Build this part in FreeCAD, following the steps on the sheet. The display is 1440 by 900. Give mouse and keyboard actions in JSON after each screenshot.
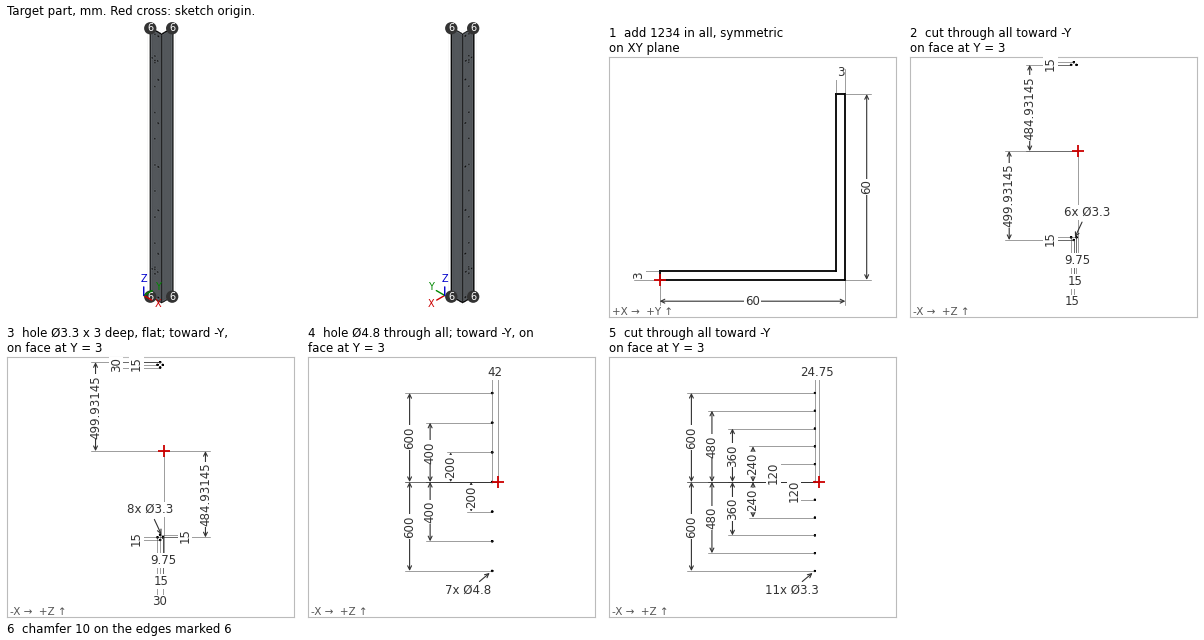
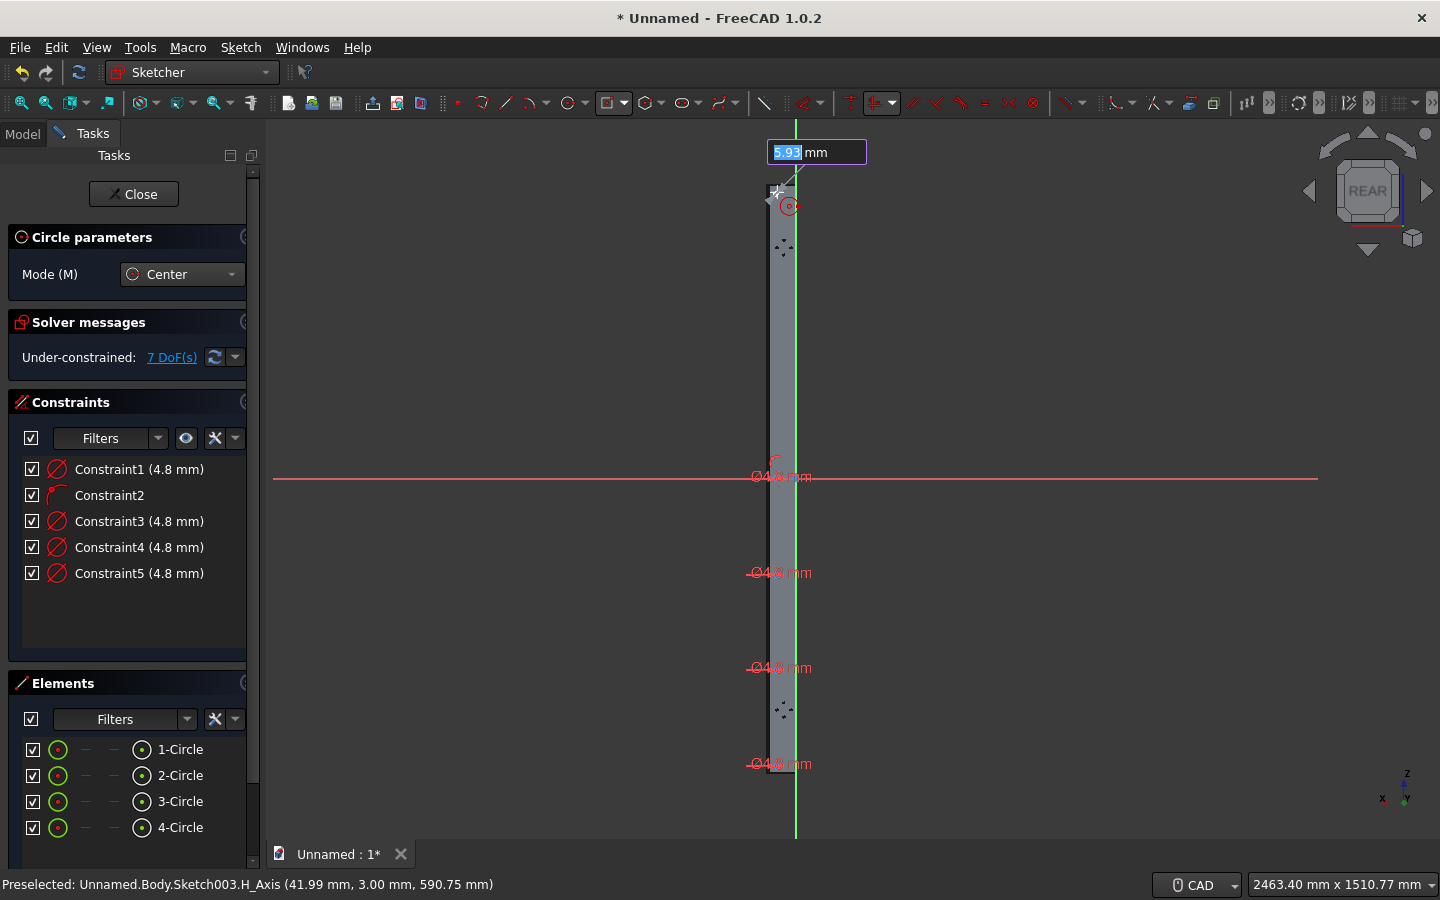
{"action": "type", "text": "4.8"}
{"action": "key", "text": "Return"}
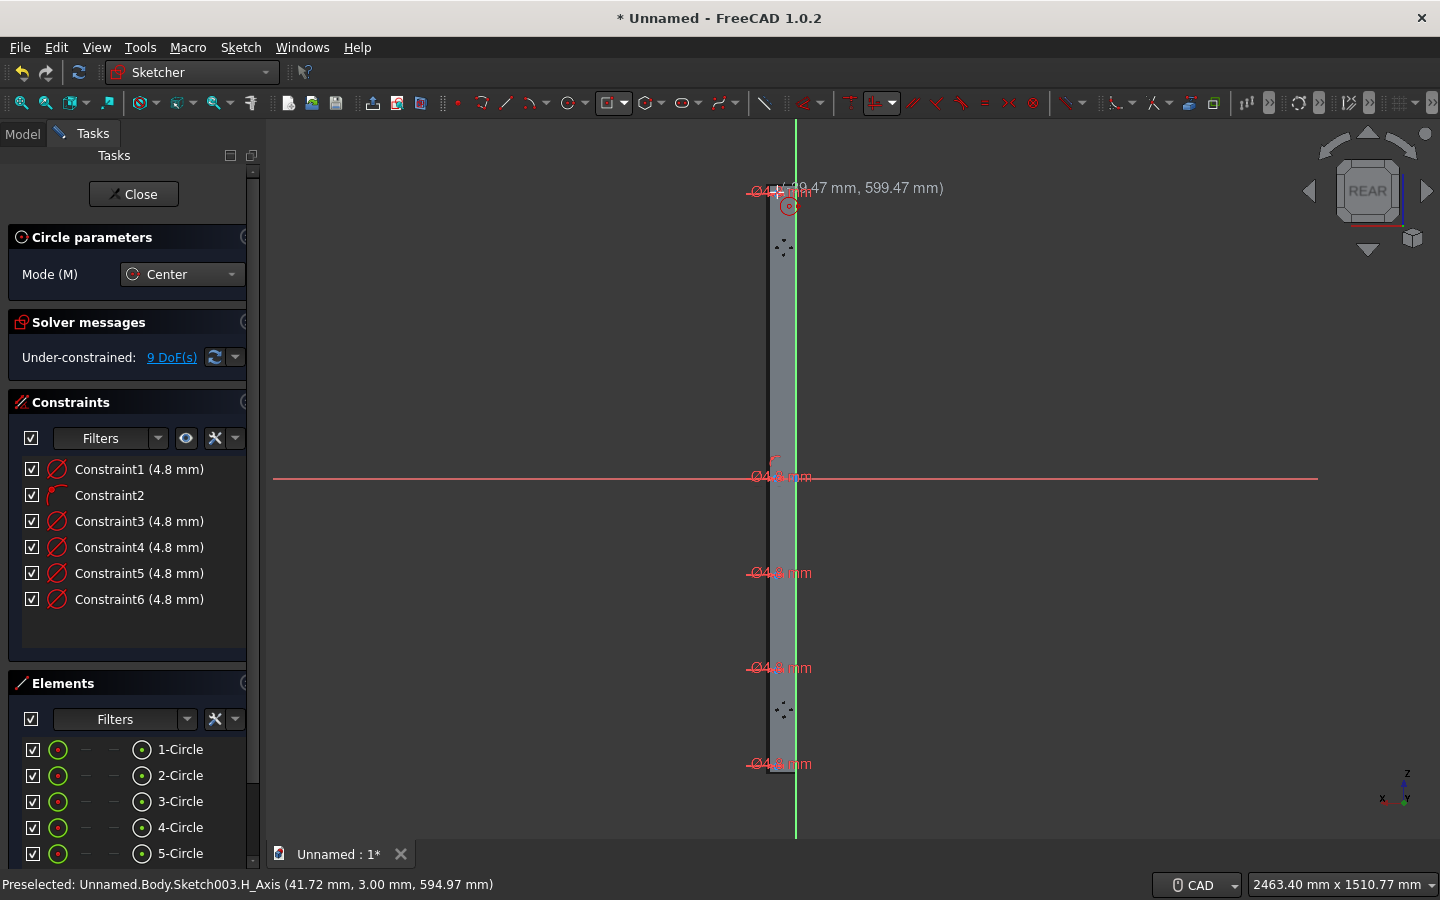
{"action": "scroll", "coordinate": [776, 288], "scroll_direction": "up", "scroll_amount": 15}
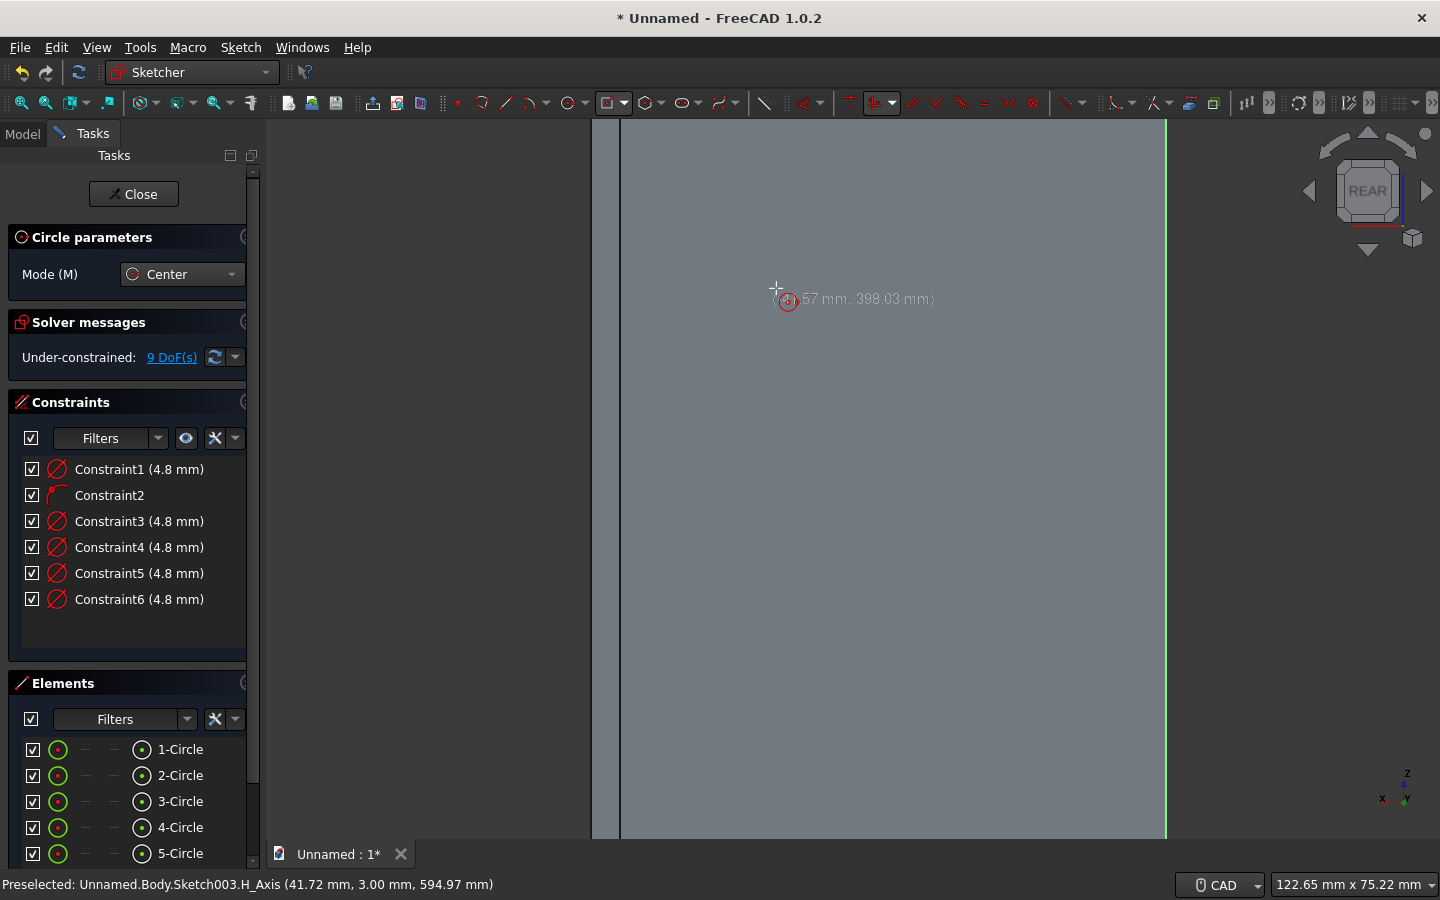
{"action": "scroll", "coordinate": [776, 289], "scroll_direction": "down", "scroll_amount": 15}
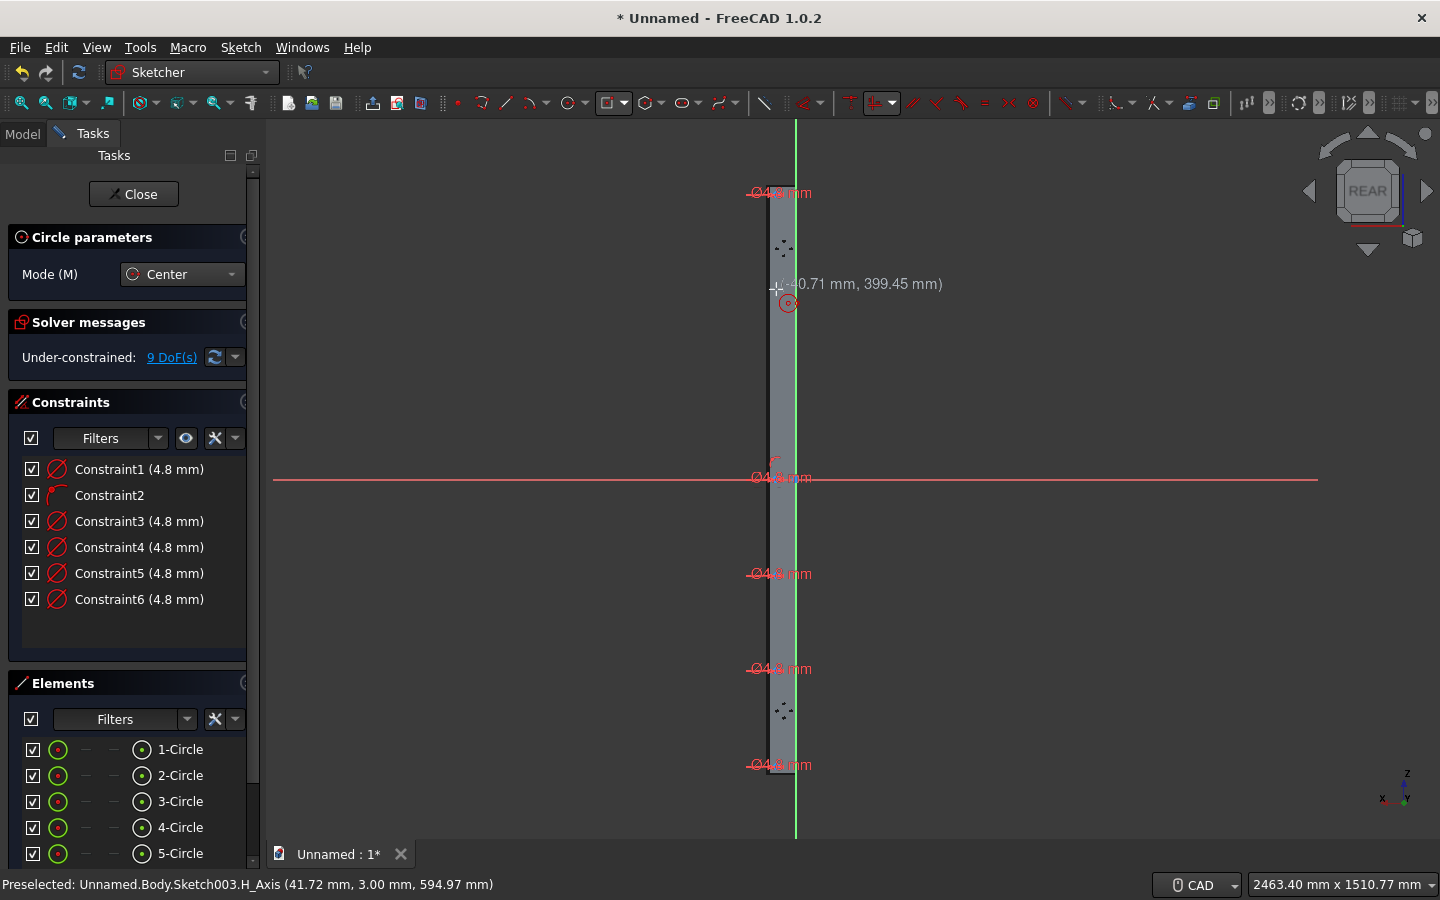
{"action": "left_click", "coordinate": [776, 289]}
{"action": "mouse_move", "coordinate": [777, 288]}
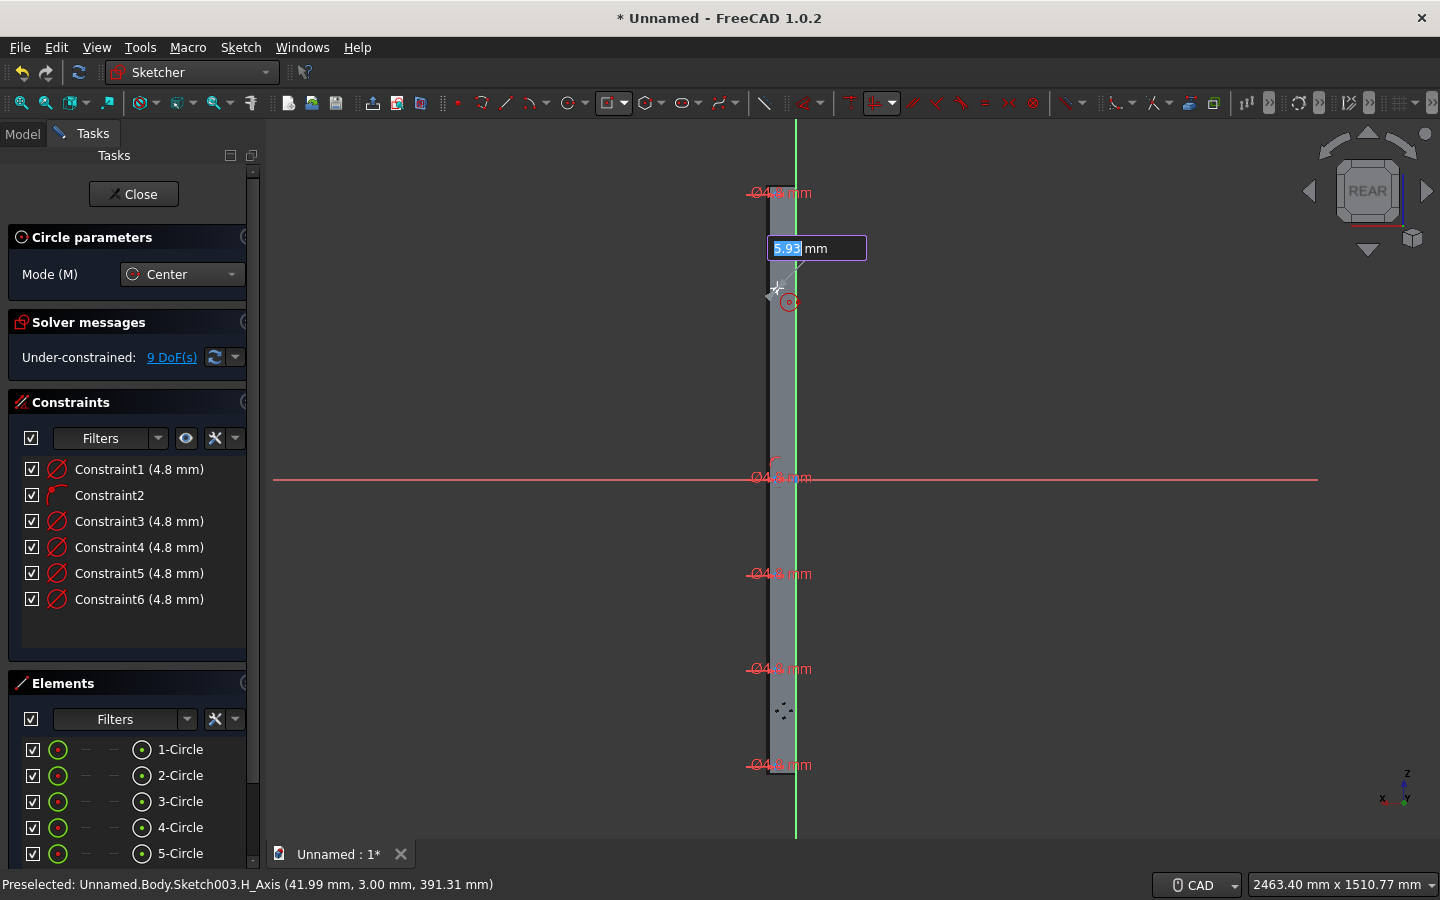
{"action": "type", "text": "4.8"}
{"action": "key", "text": "Return"}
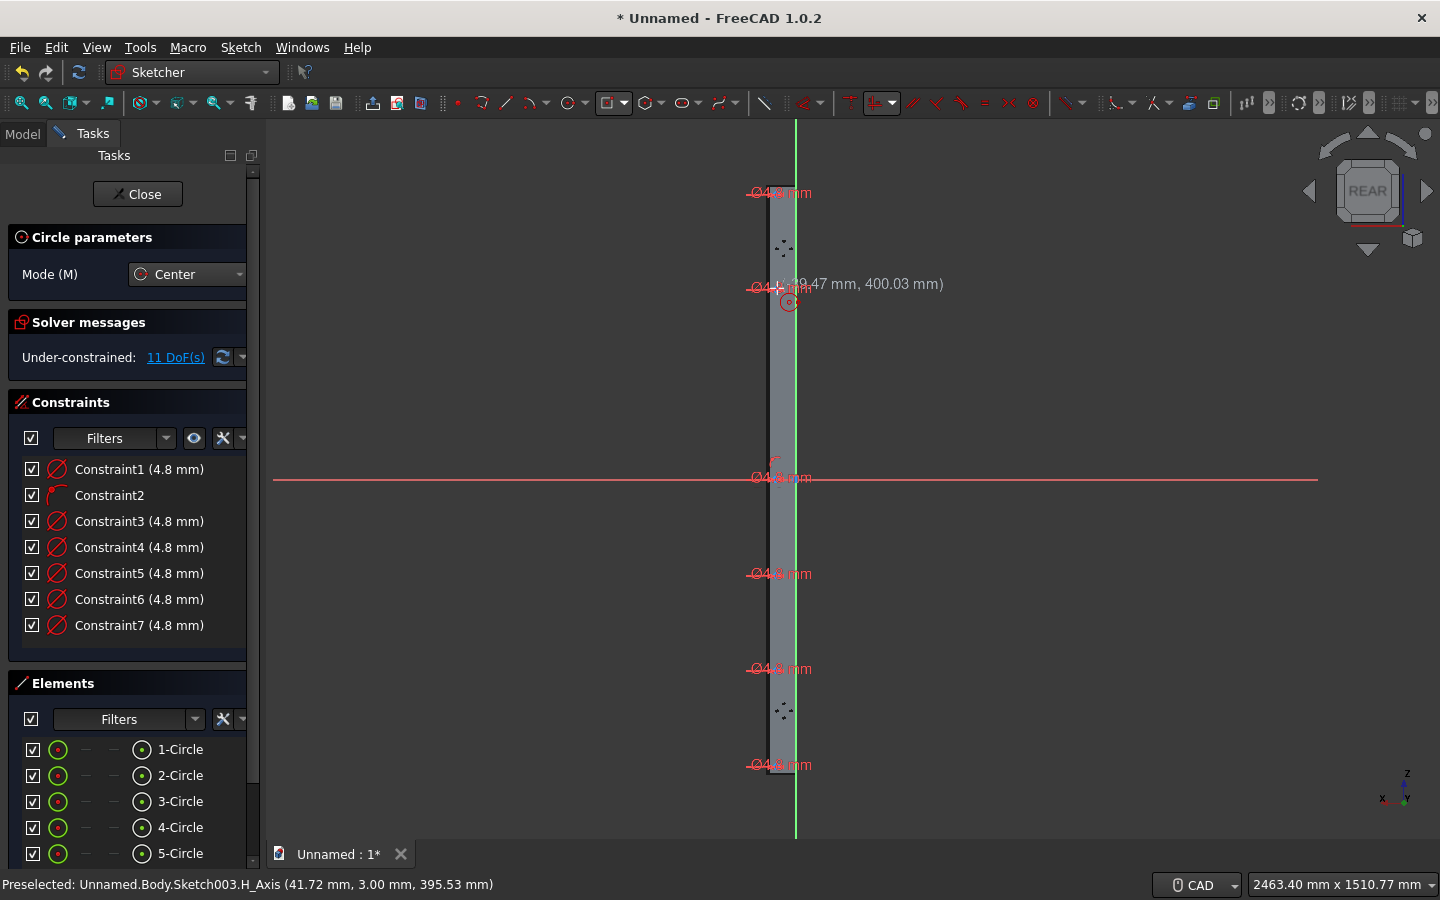
{"action": "scroll", "coordinate": [776, 384], "scroll_direction": "up", "scroll_amount": 15}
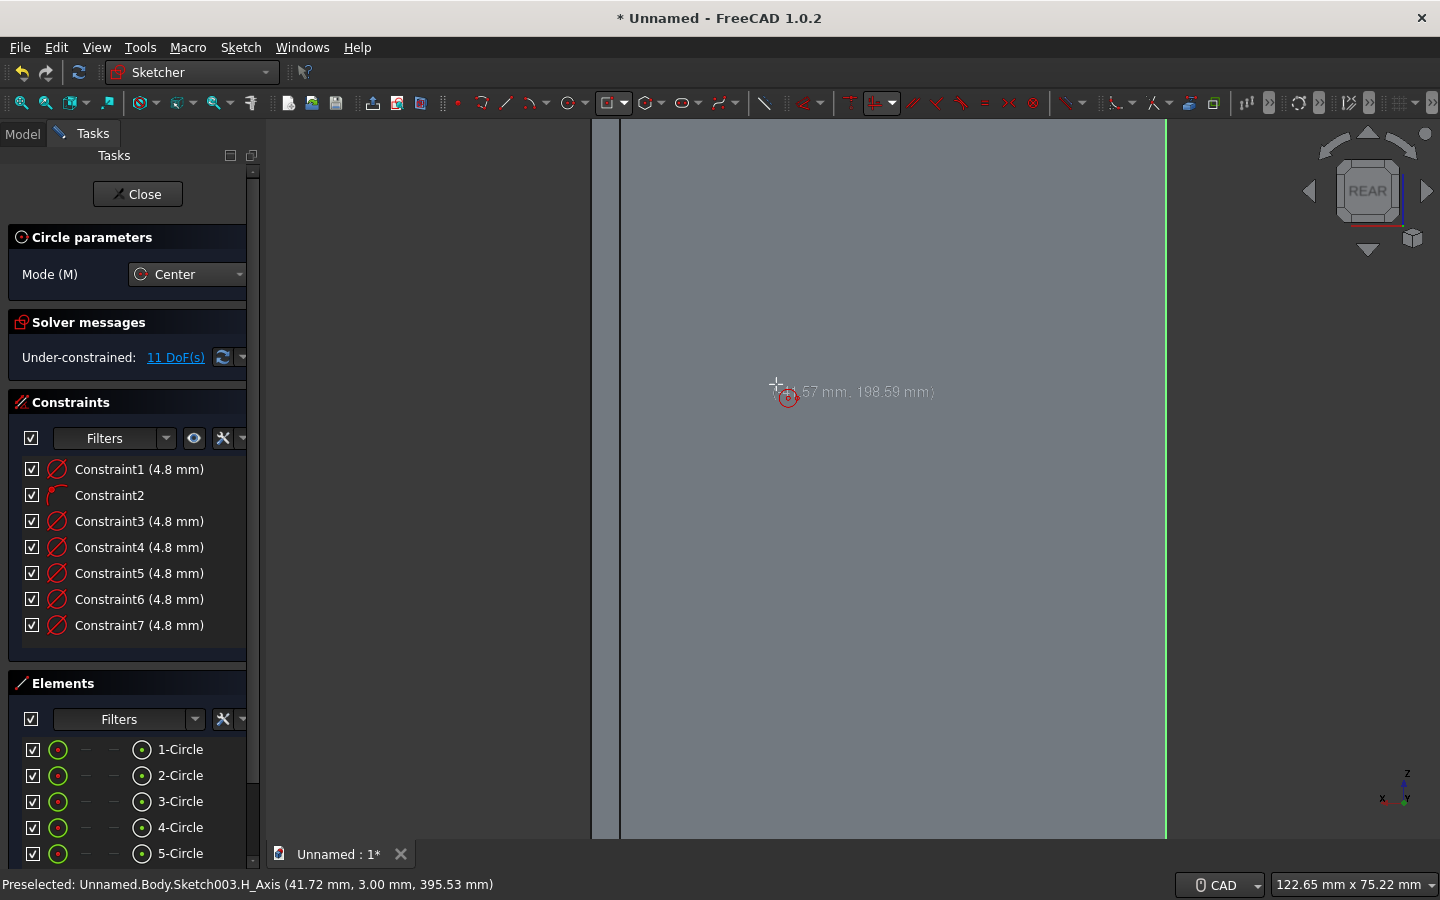
{"action": "scroll", "coordinate": [776, 384], "scroll_direction": "down", "scroll_amount": 15}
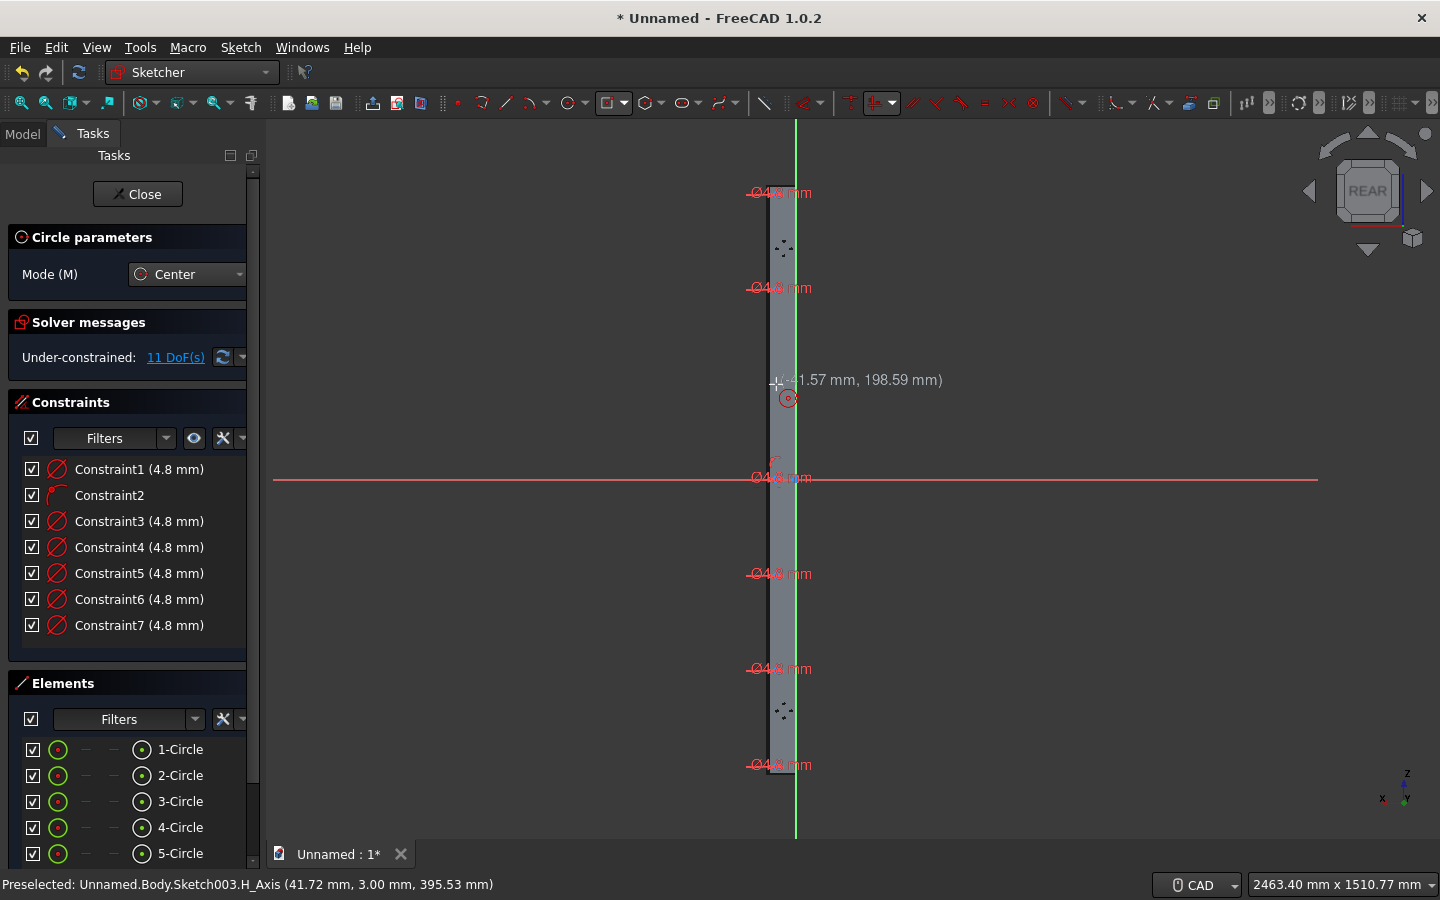
{"action": "left_click", "coordinate": [776, 384]}
{"action": "mouse_move", "coordinate": [777, 384]}